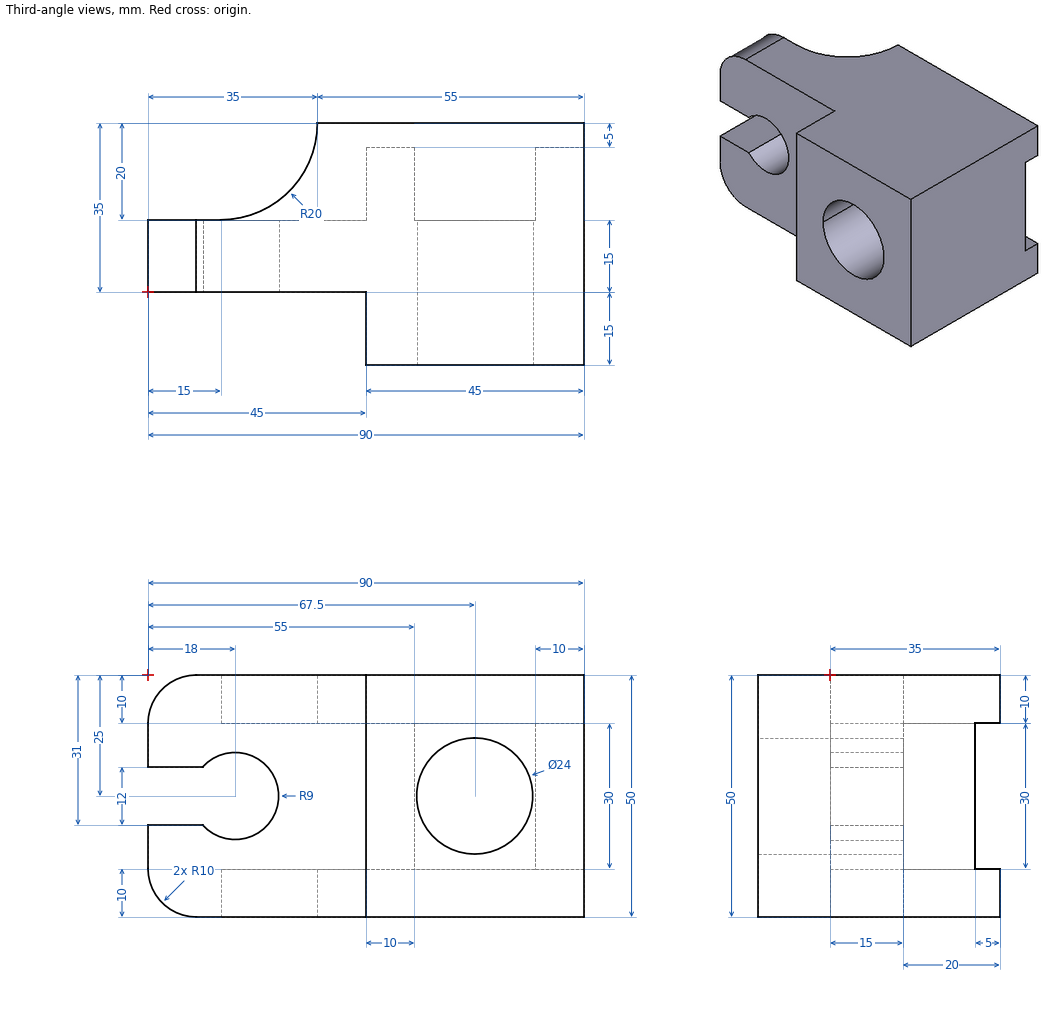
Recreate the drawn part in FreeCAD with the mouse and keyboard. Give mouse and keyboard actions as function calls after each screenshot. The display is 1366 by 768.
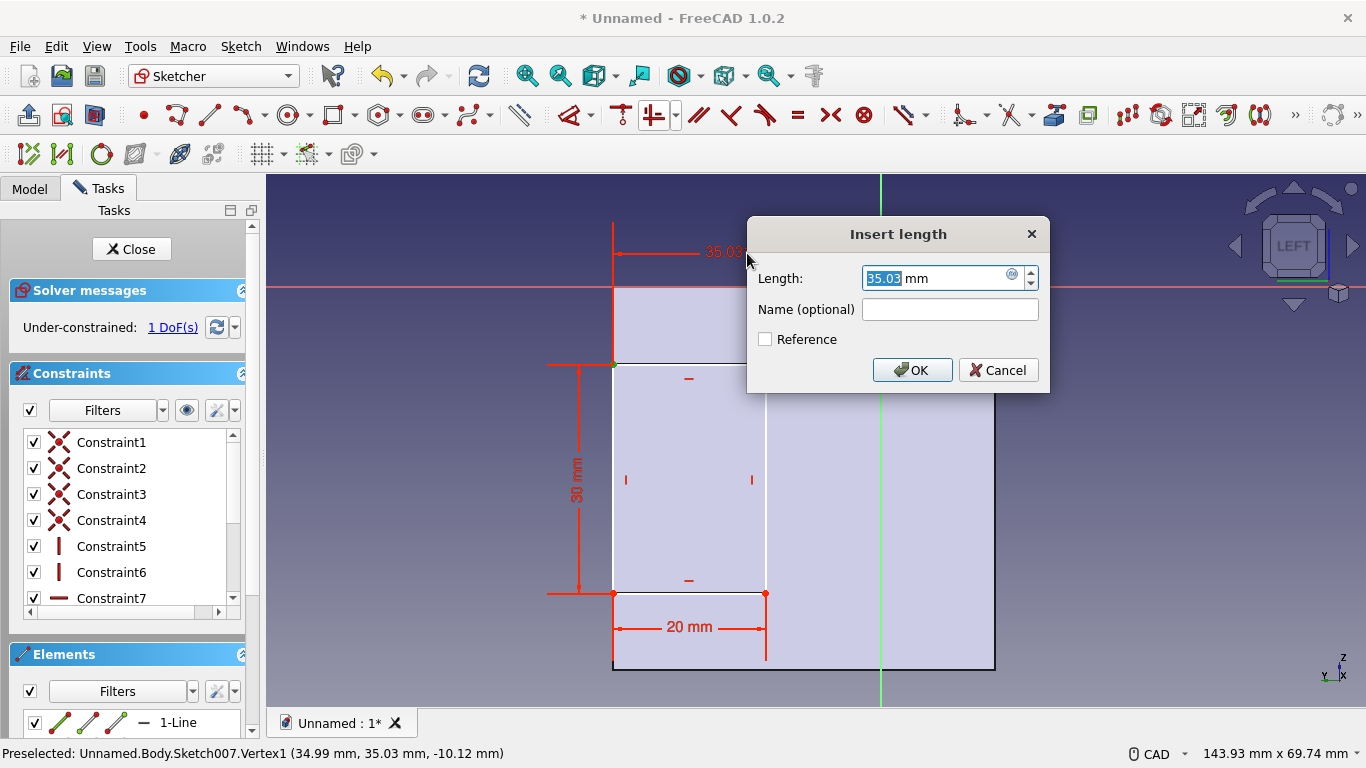
text(35)
key(Return)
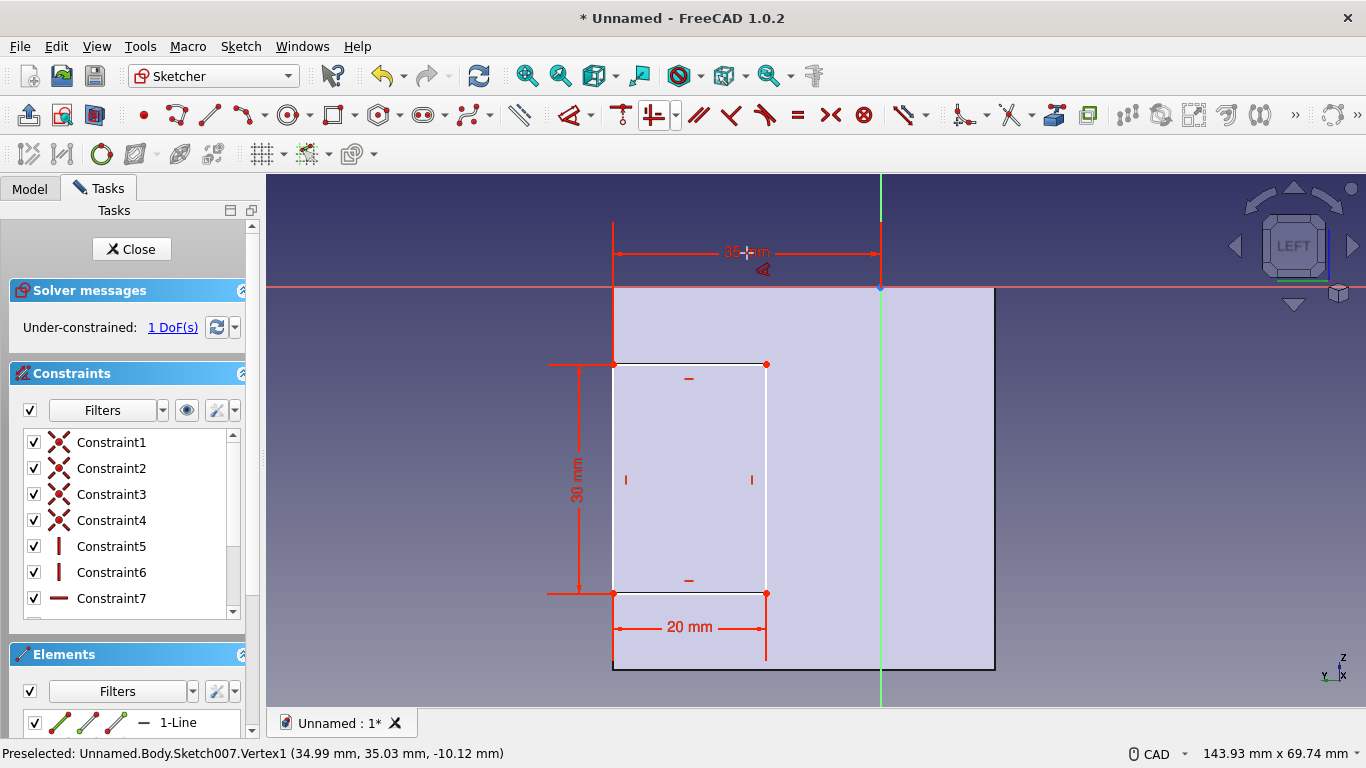
click(613, 365)
click(915, 326)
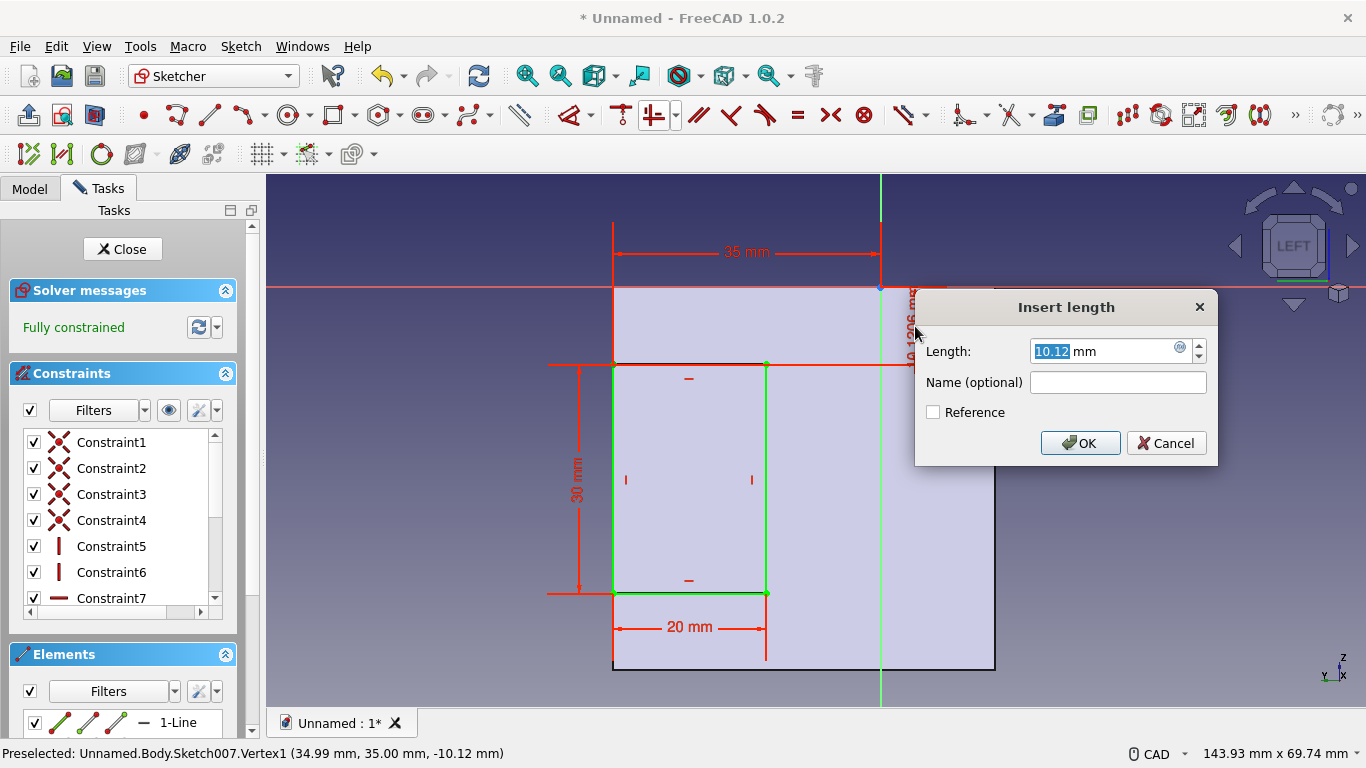
text(10)
key(Return)
key(Escape)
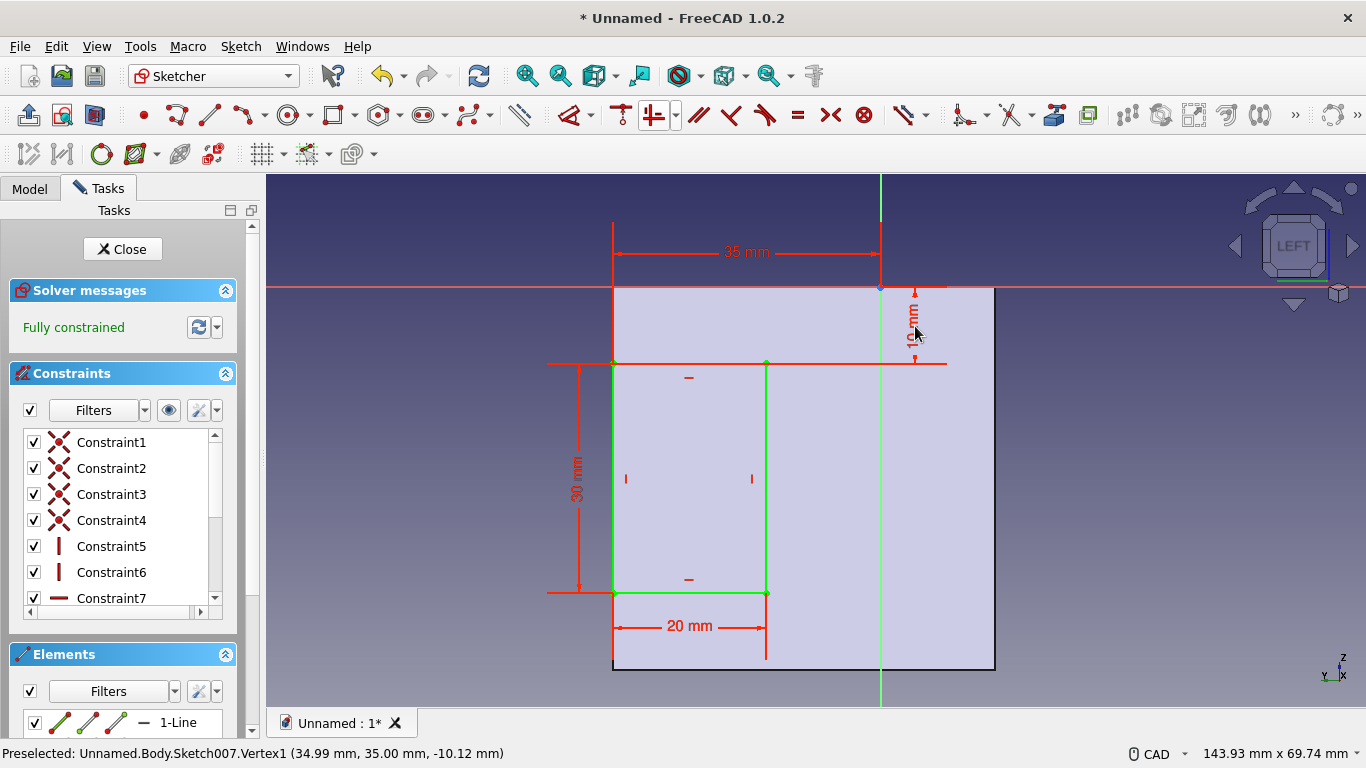
click(123, 249)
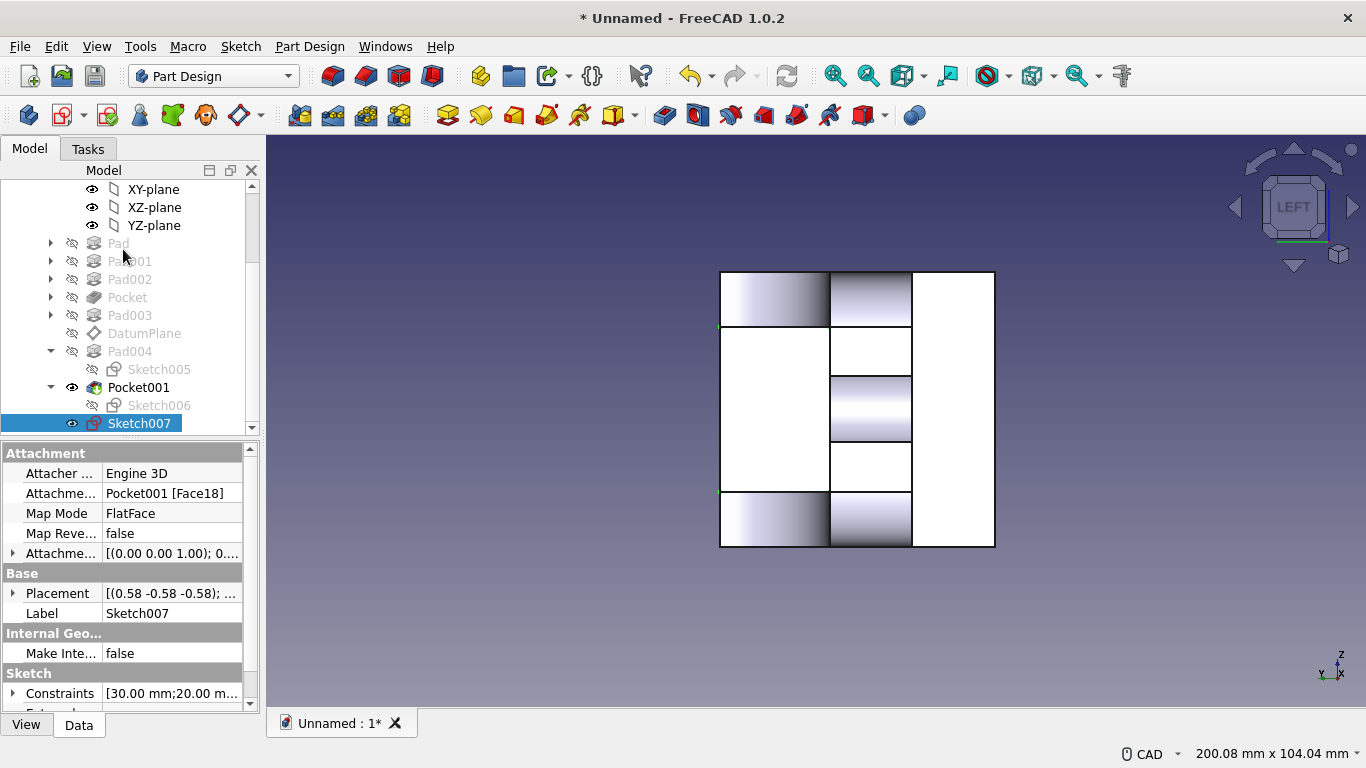
click(665, 116)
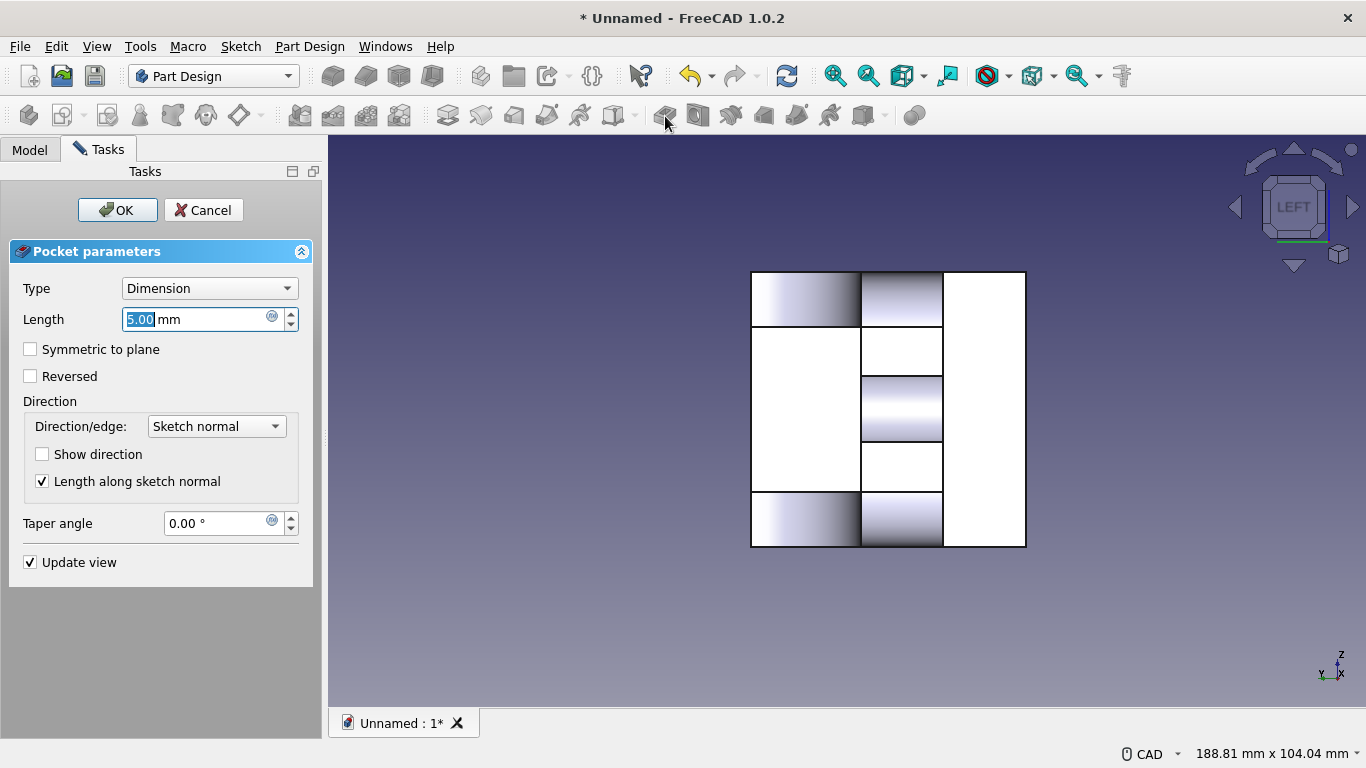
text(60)
key(Tab)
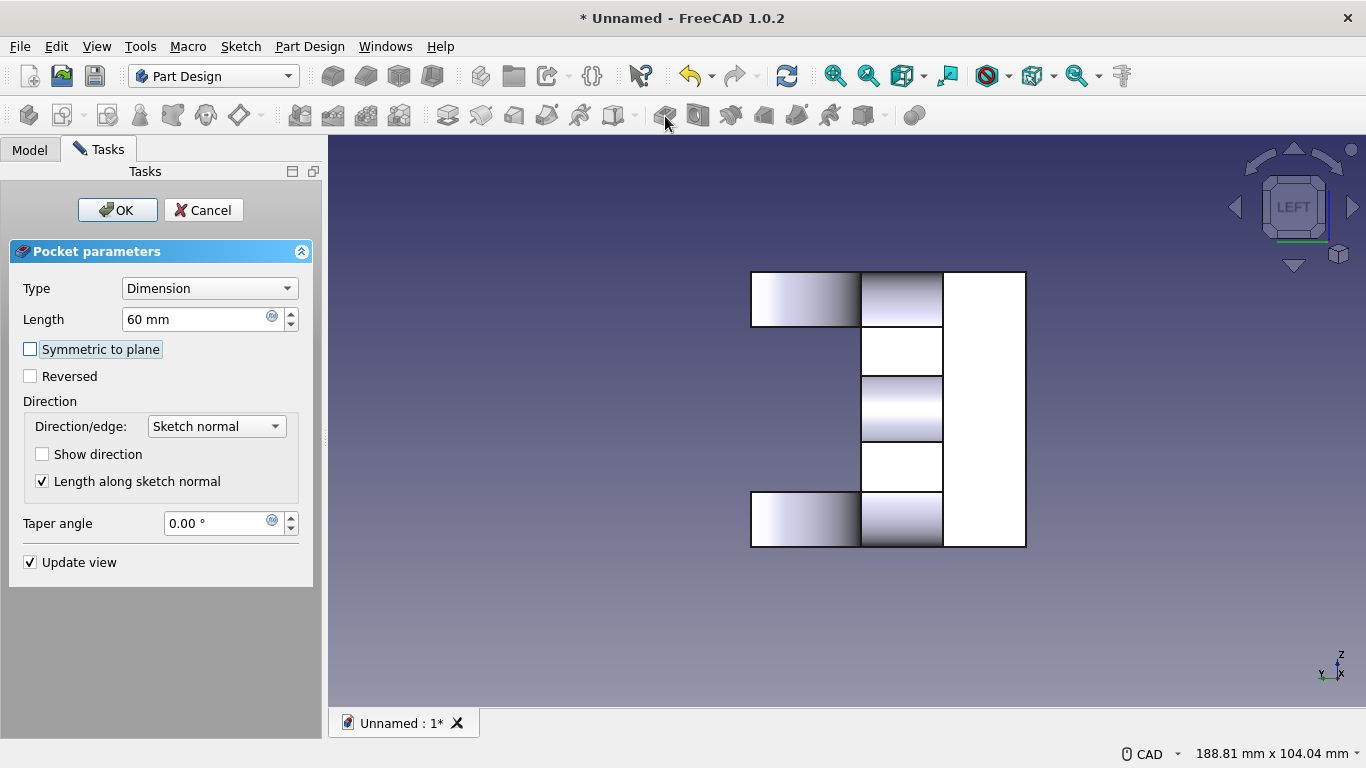
click(118, 210)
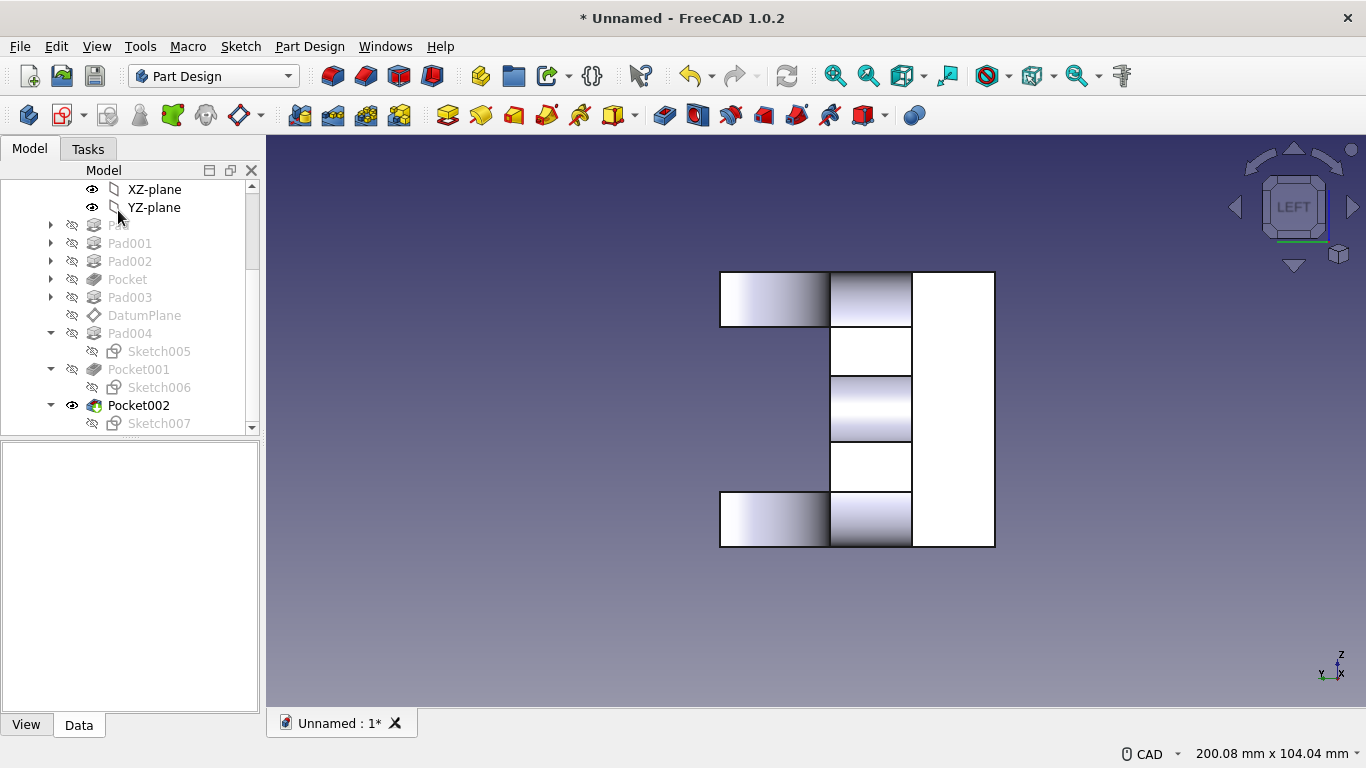
key(0)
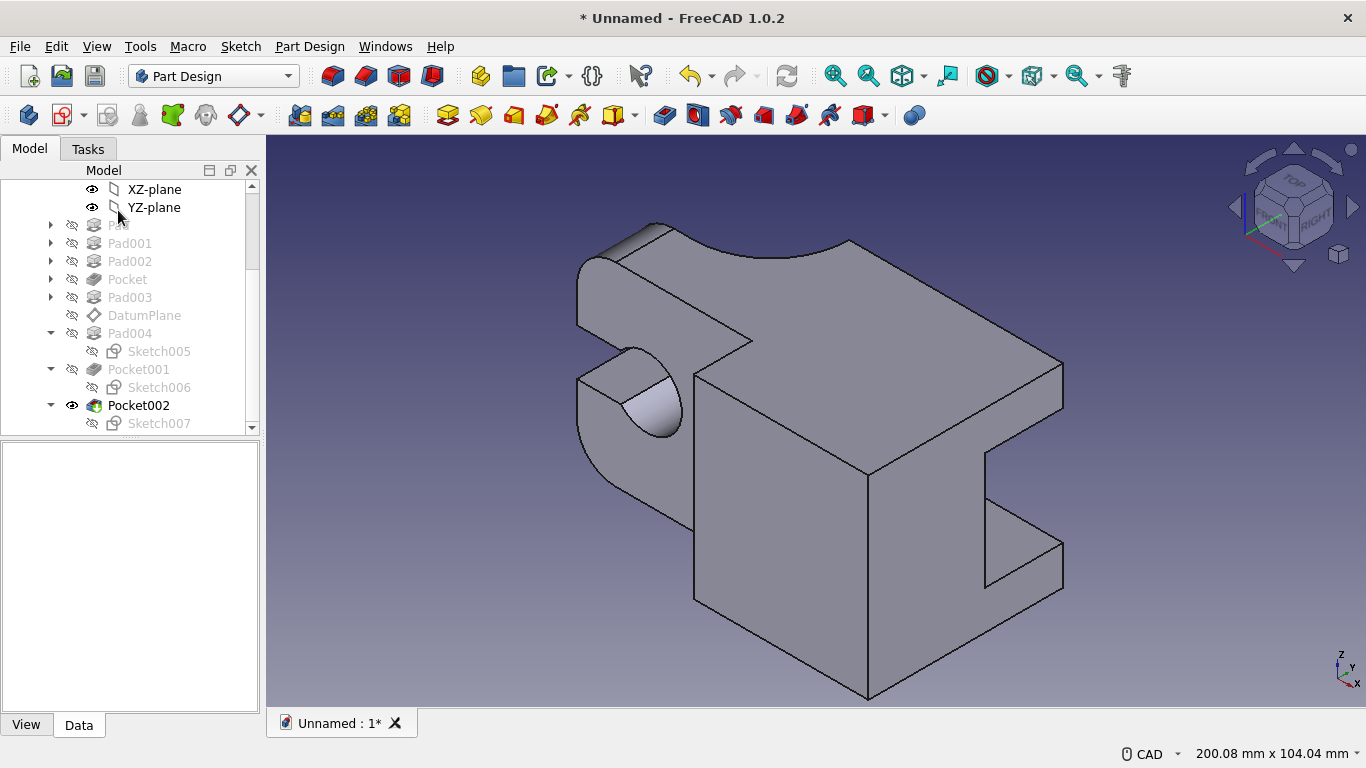
click(938, 515)